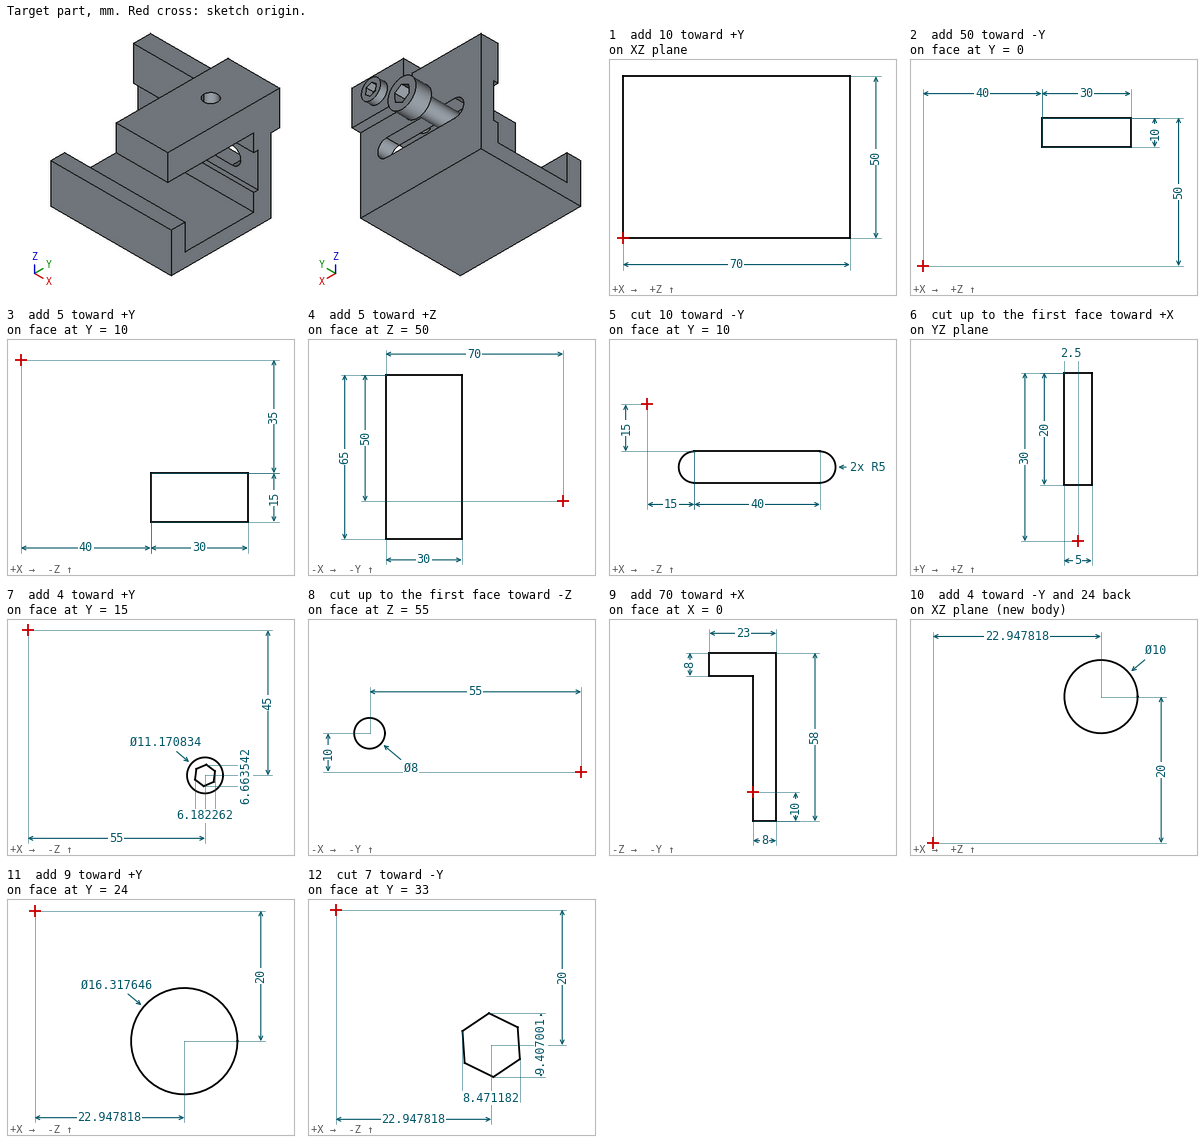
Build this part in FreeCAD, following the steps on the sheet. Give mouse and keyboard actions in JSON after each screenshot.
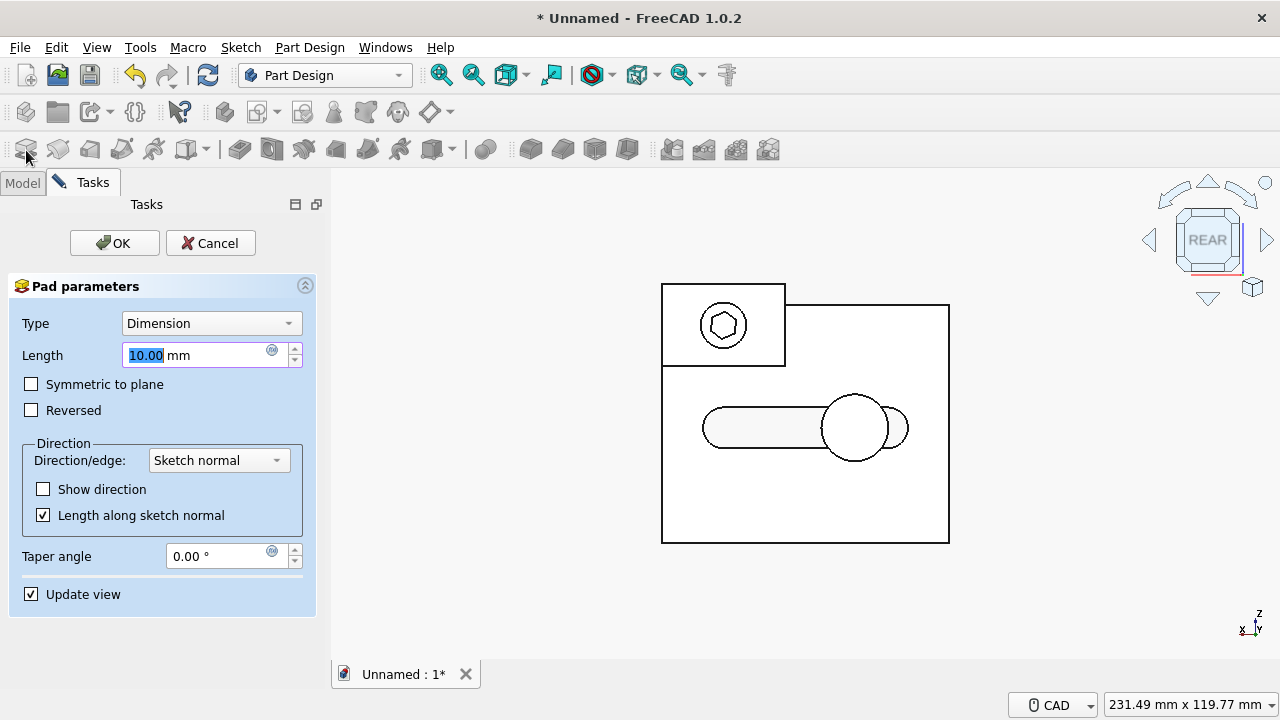
{"action": "type", "text": "9"}
{"action": "key", "text": "Tab"}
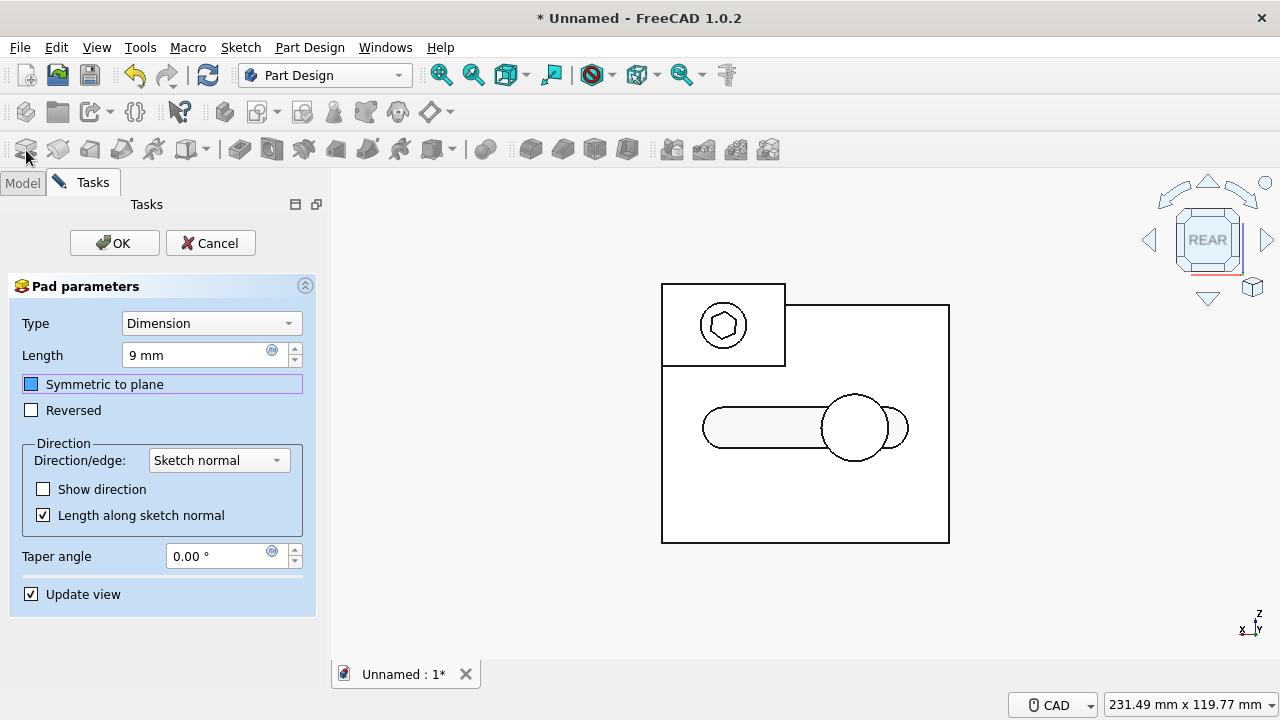
{"action": "left_click", "coordinate": [115, 243]}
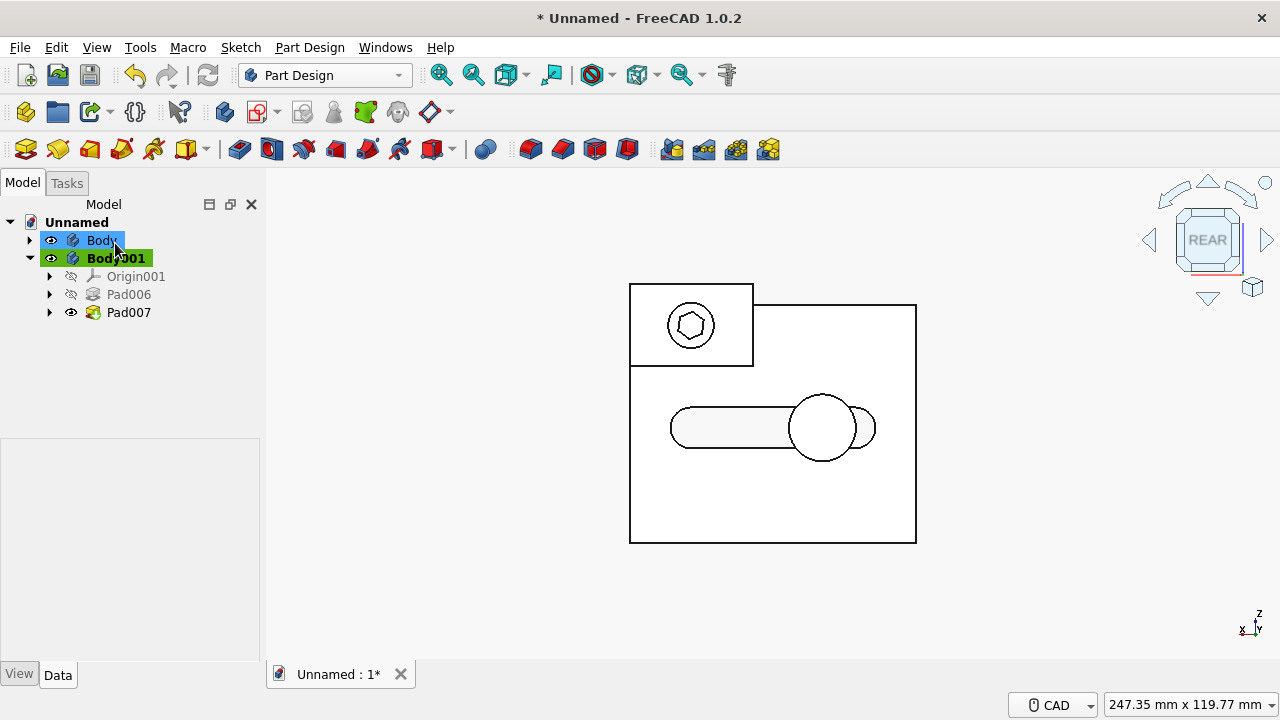
{"action": "left_click", "coordinate": [442, 76]}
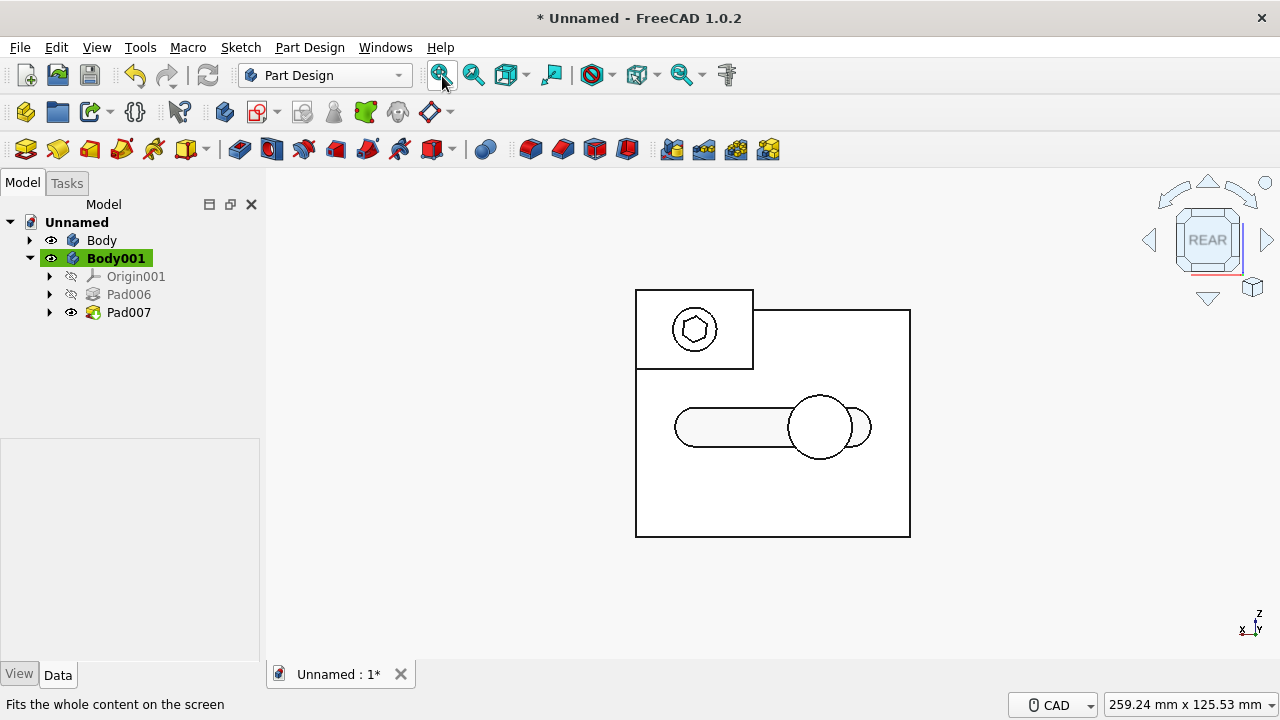
{"action": "left_click", "coordinate": [820, 426]}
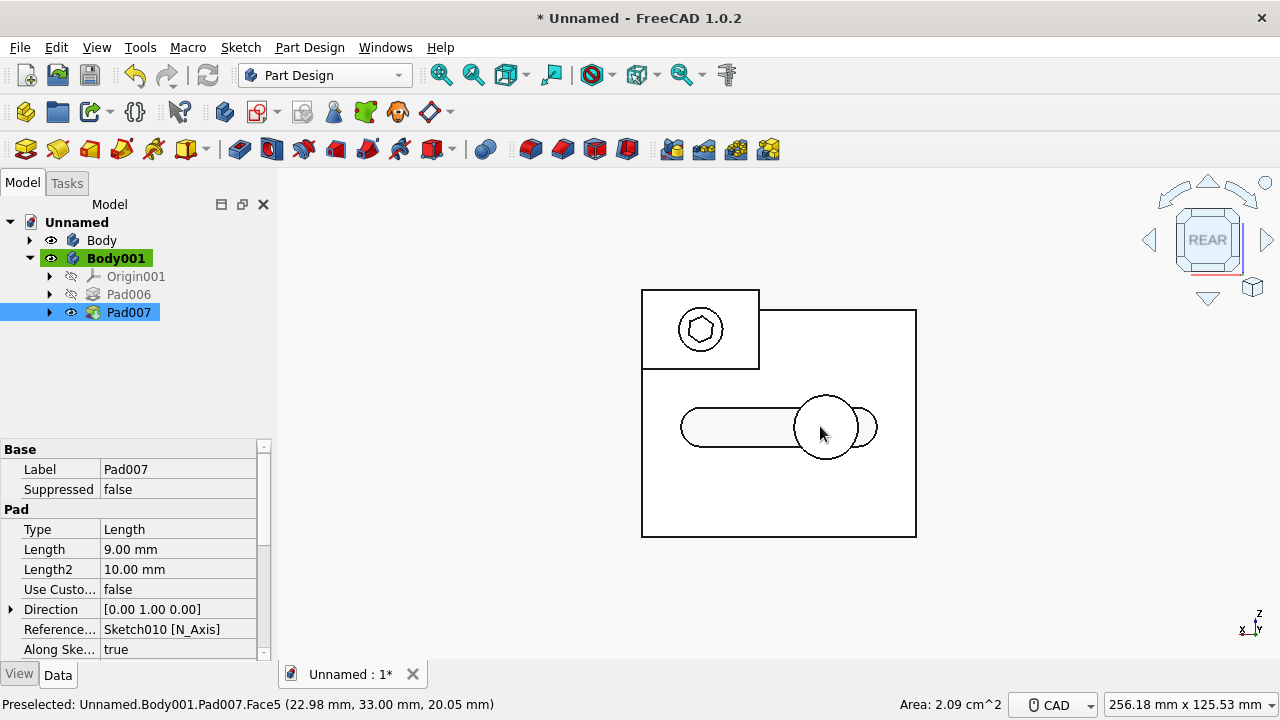
{"action": "left_click", "coordinate": [258, 112]}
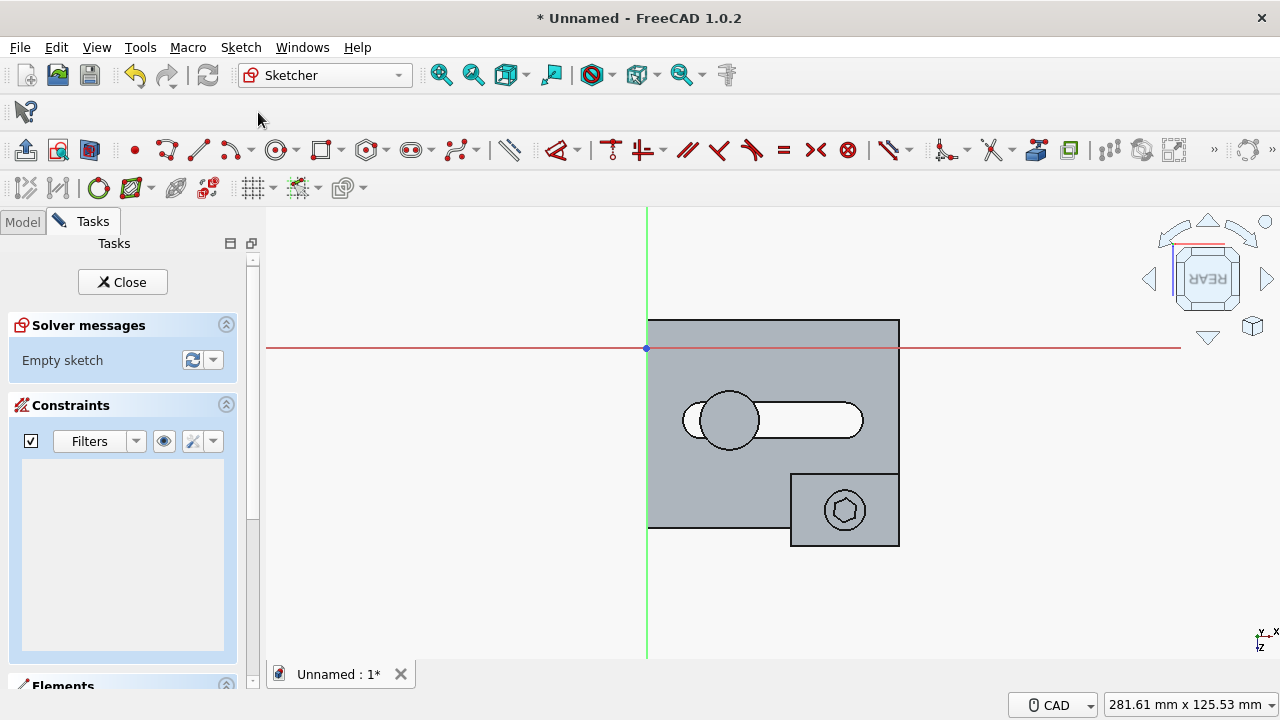
{"action": "scroll", "coordinate": [733, 419], "scroll_direction": "up", "scroll_amount": 11}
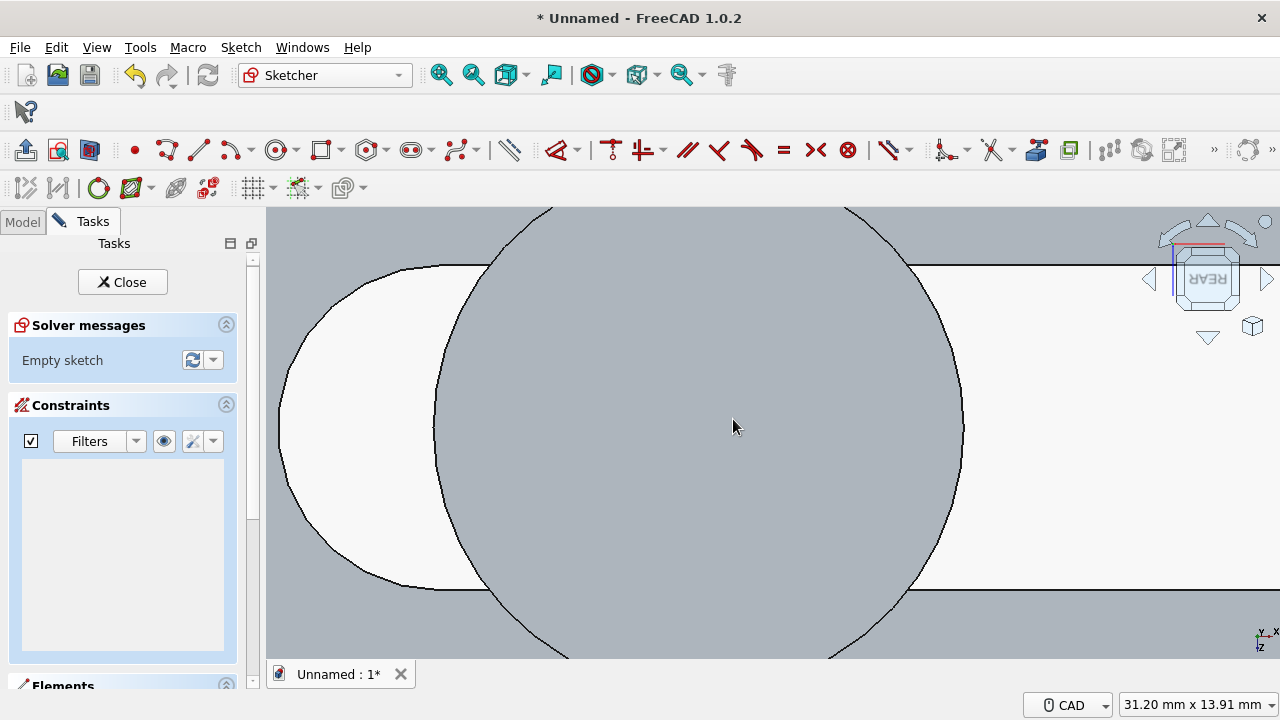
{"action": "left_click", "coordinate": [366, 150]}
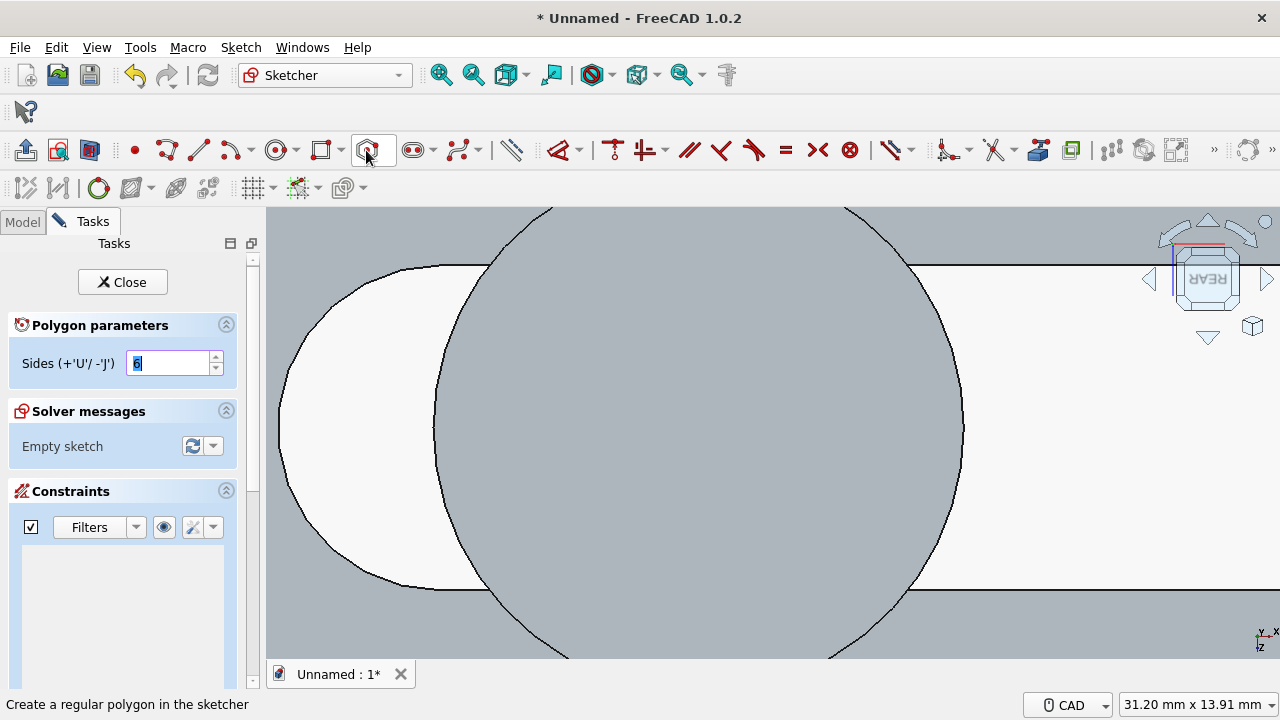
{"action": "left_click", "coordinate": [699, 428]}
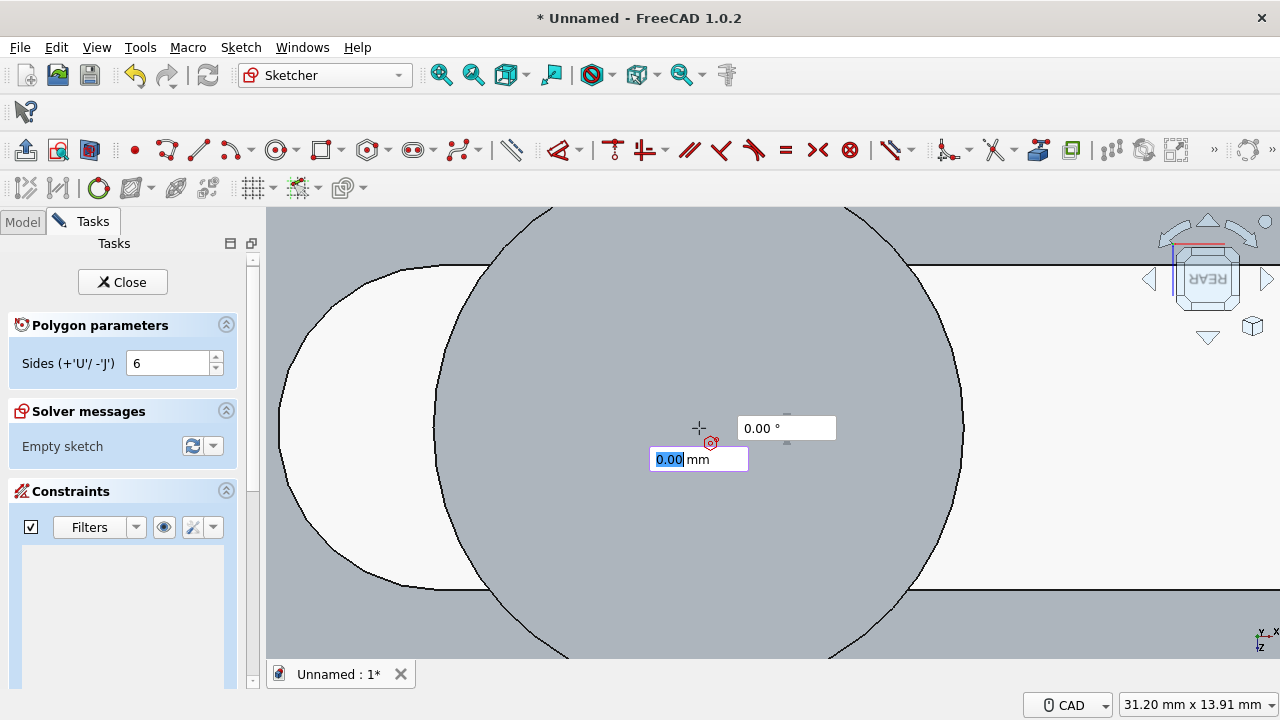
{"action": "left_click", "coordinate": [709, 581]}
{"action": "key", "text": "Escape"}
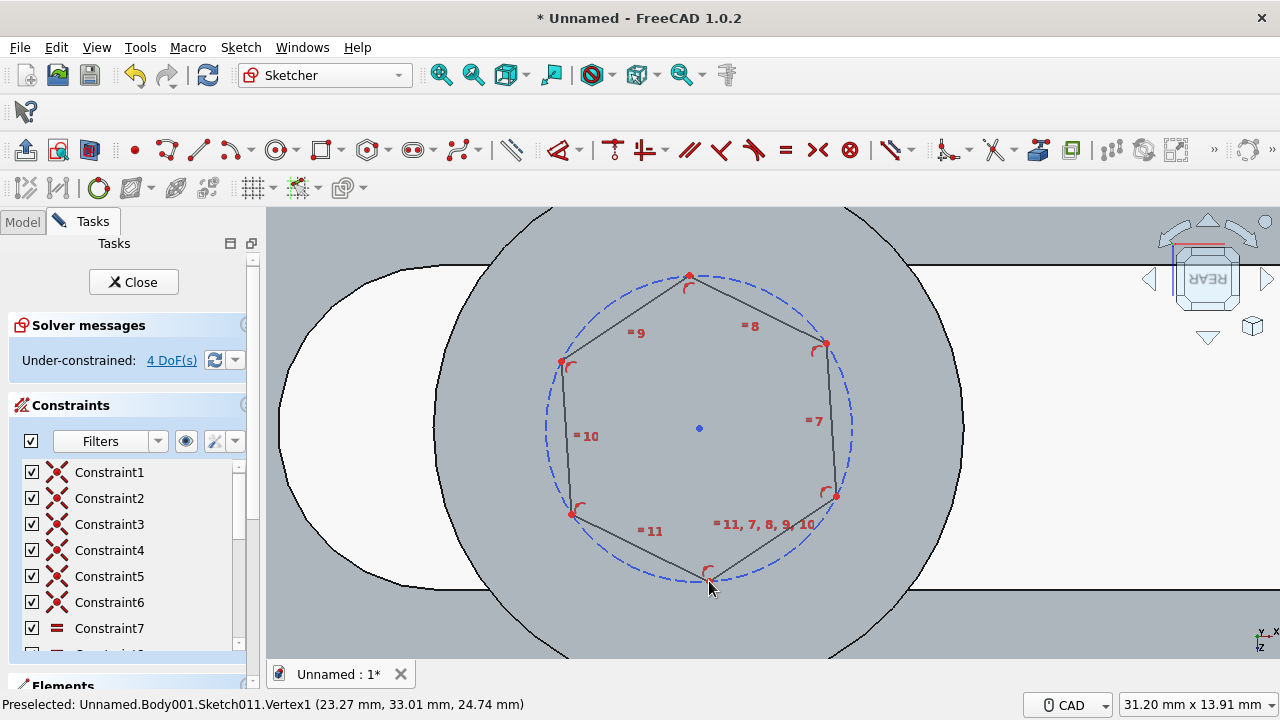
{"action": "left_click", "coordinate": [558, 150]}